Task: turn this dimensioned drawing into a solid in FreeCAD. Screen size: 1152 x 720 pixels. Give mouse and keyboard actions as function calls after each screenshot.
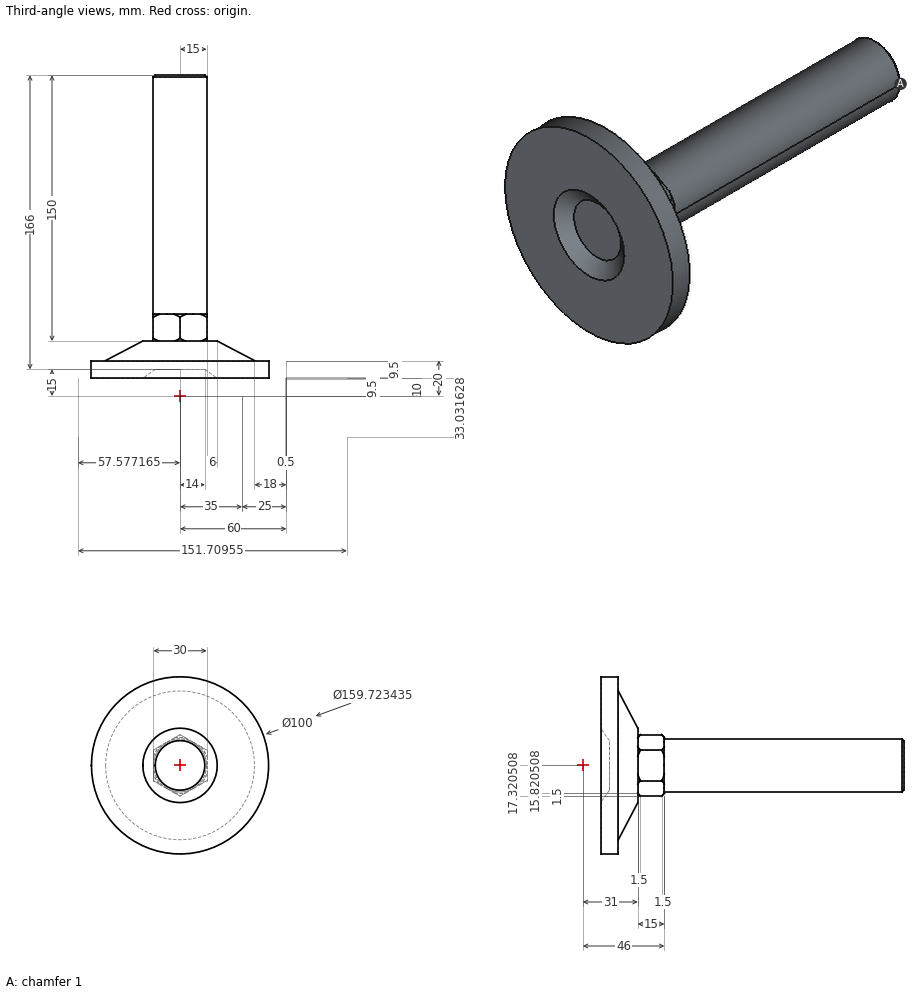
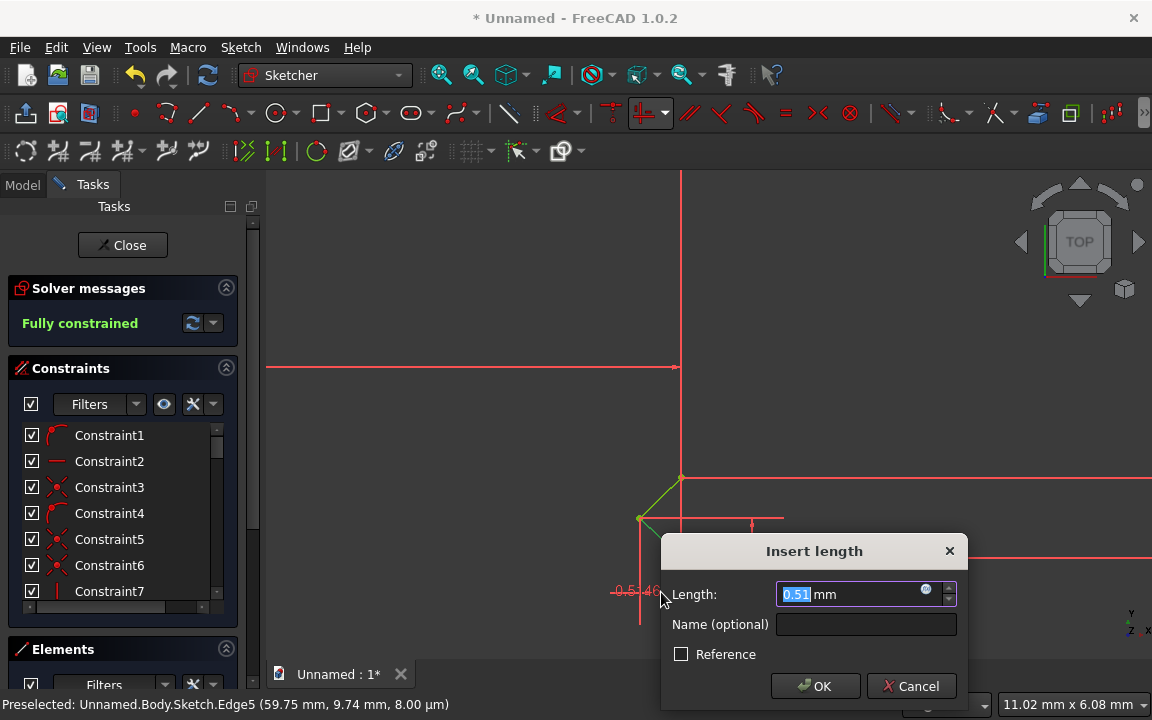
text(0.5)
key(Return)
key(Escape)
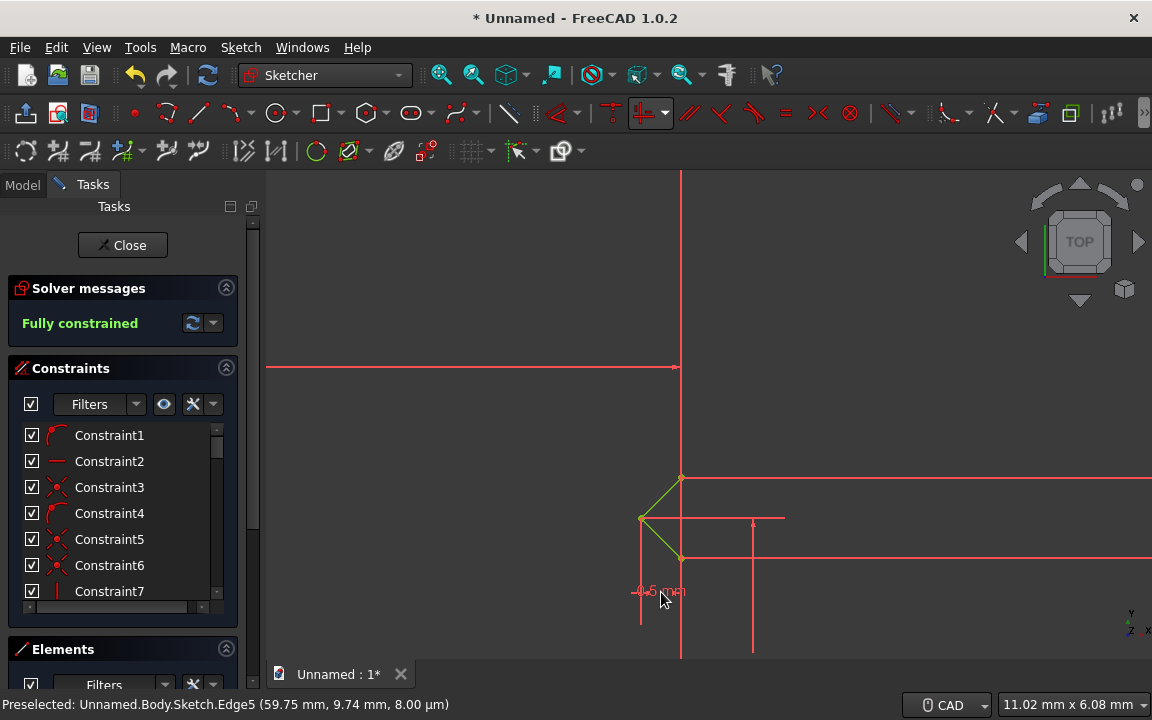
click(123, 245)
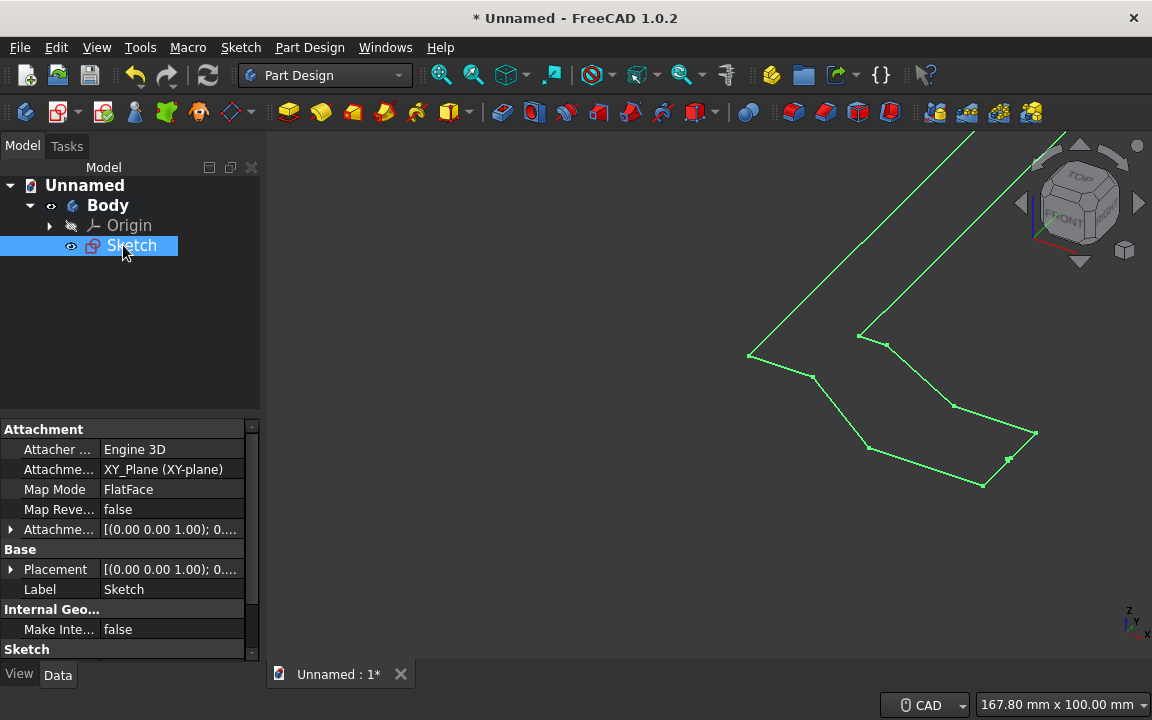
click(322, 112)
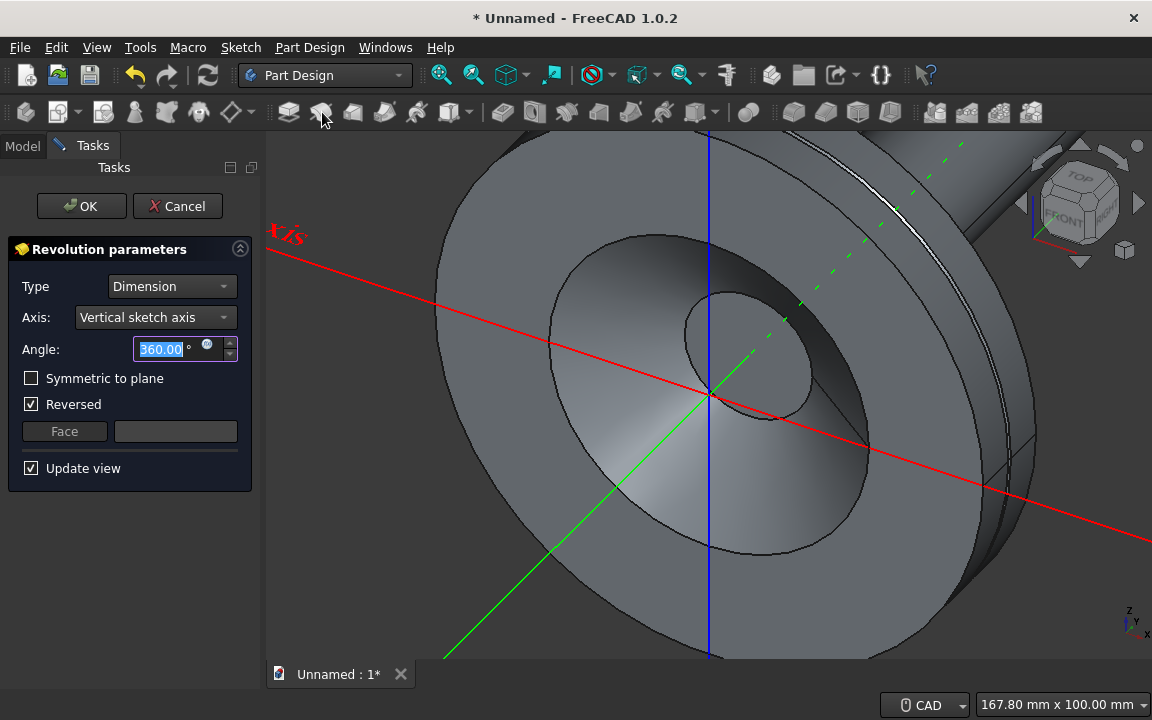
click(82, 206)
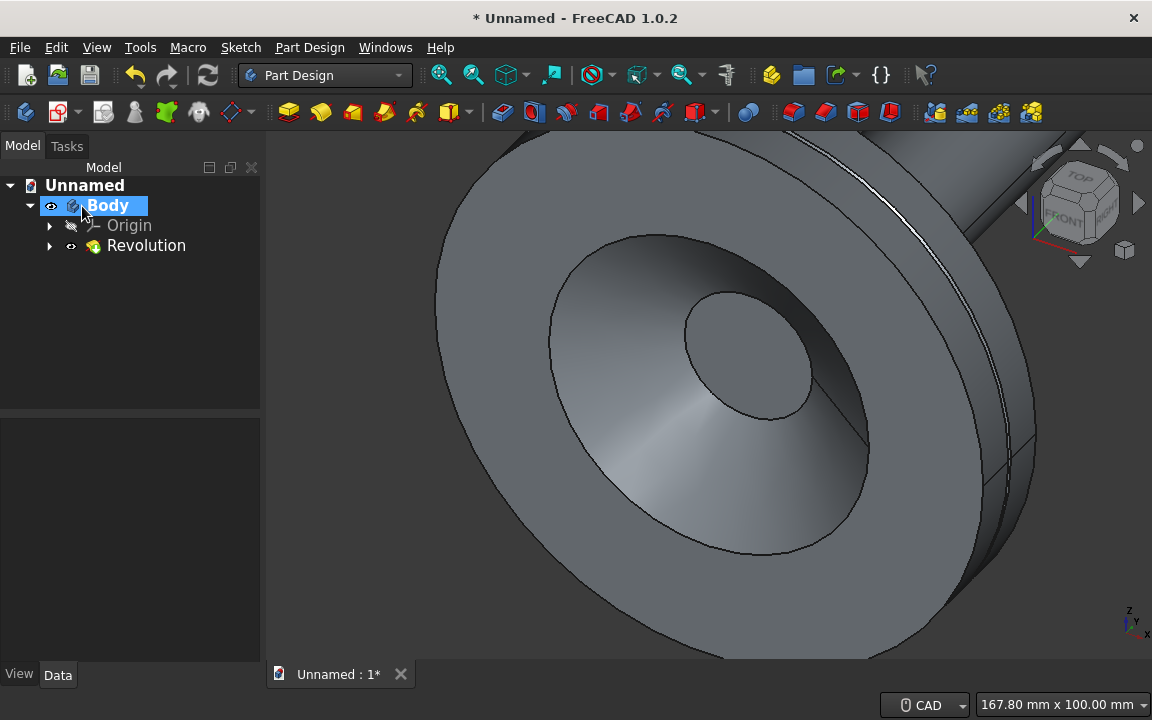
click(442, 76)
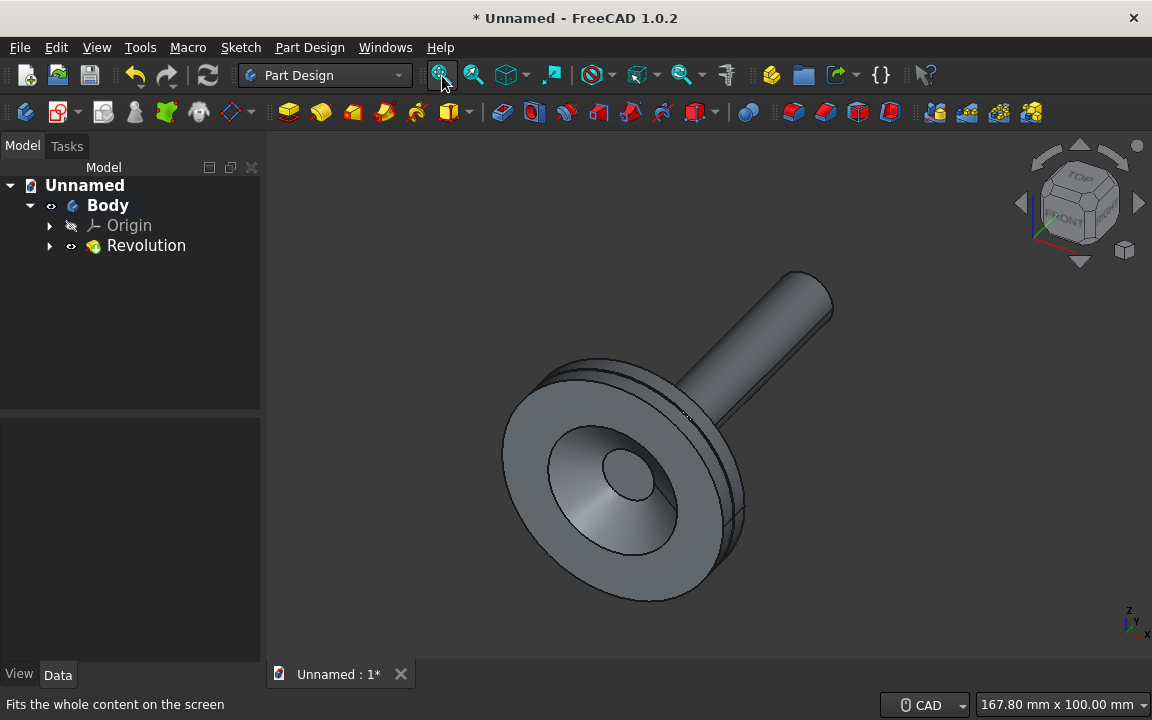
key(4)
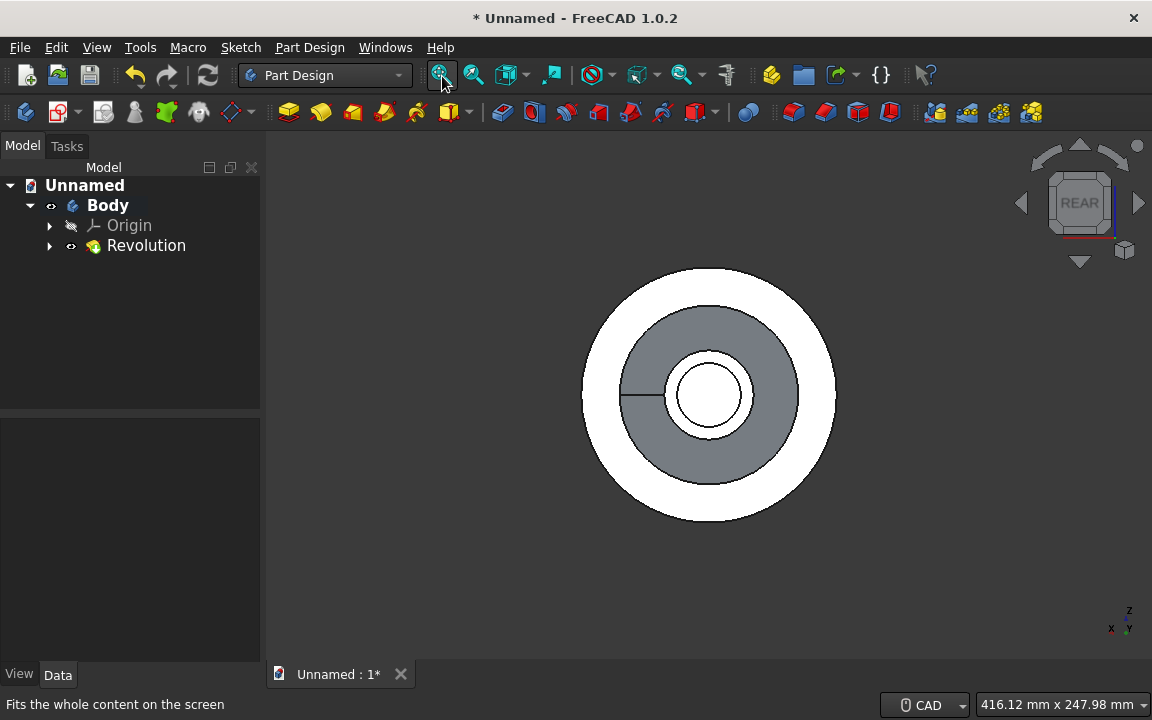
scroll(671, 394, up, 4)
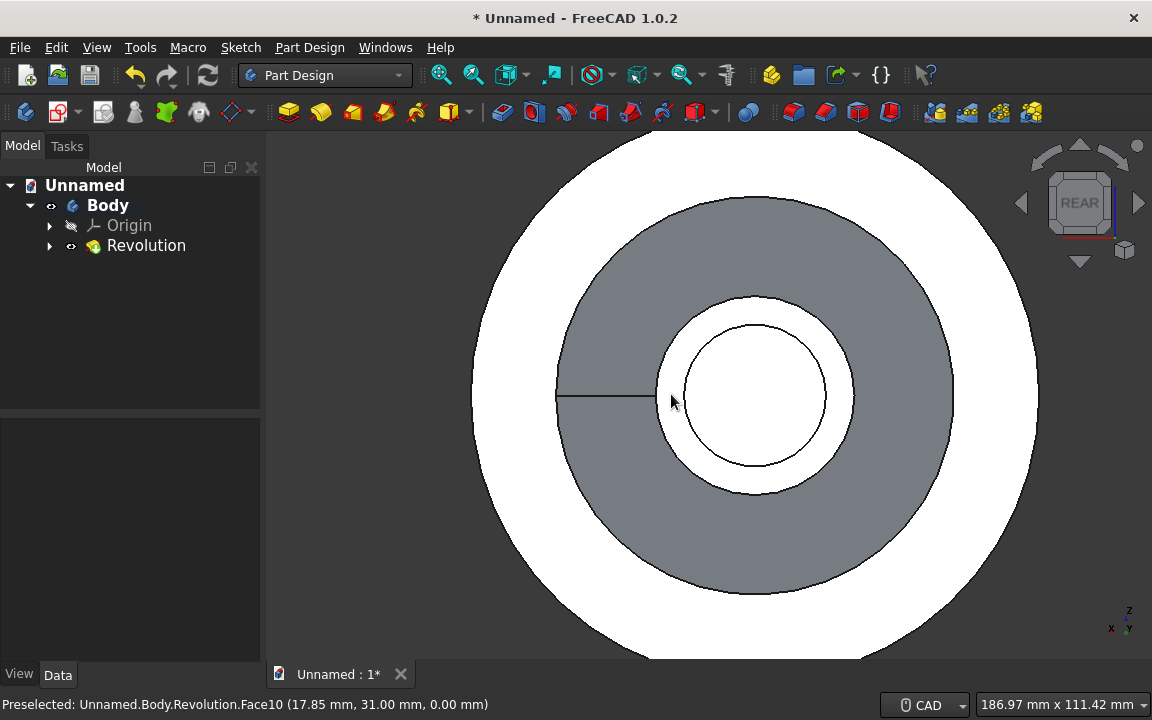
click(670, 395)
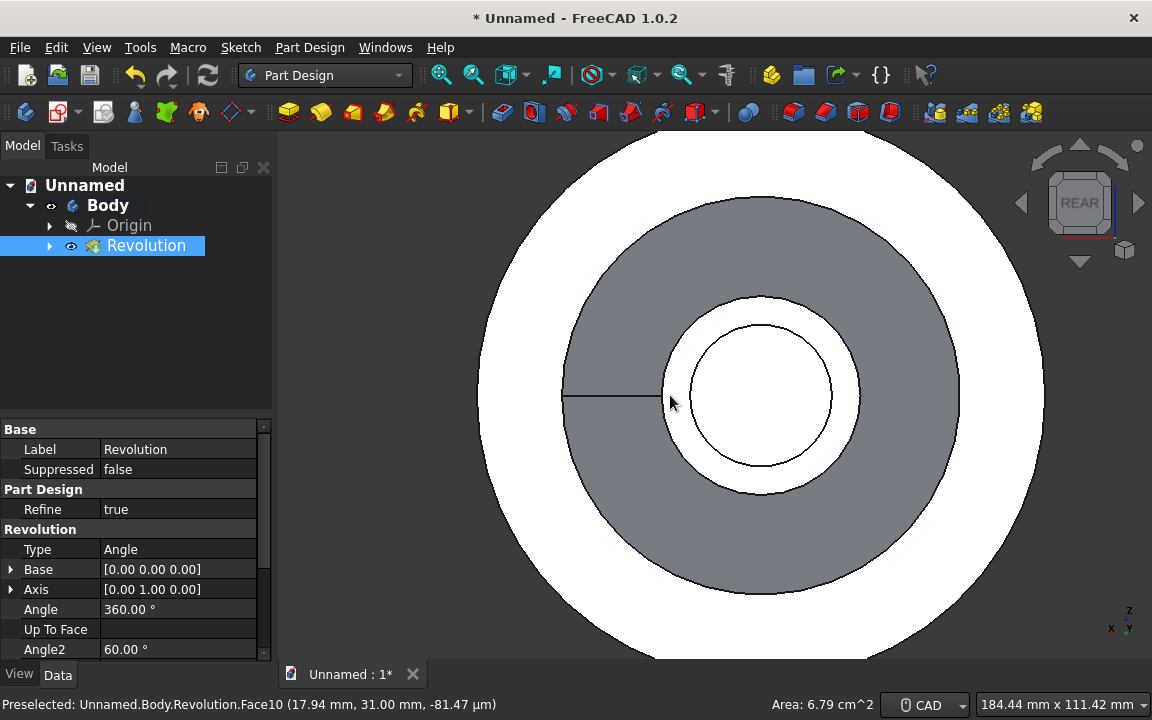
click(58, 112)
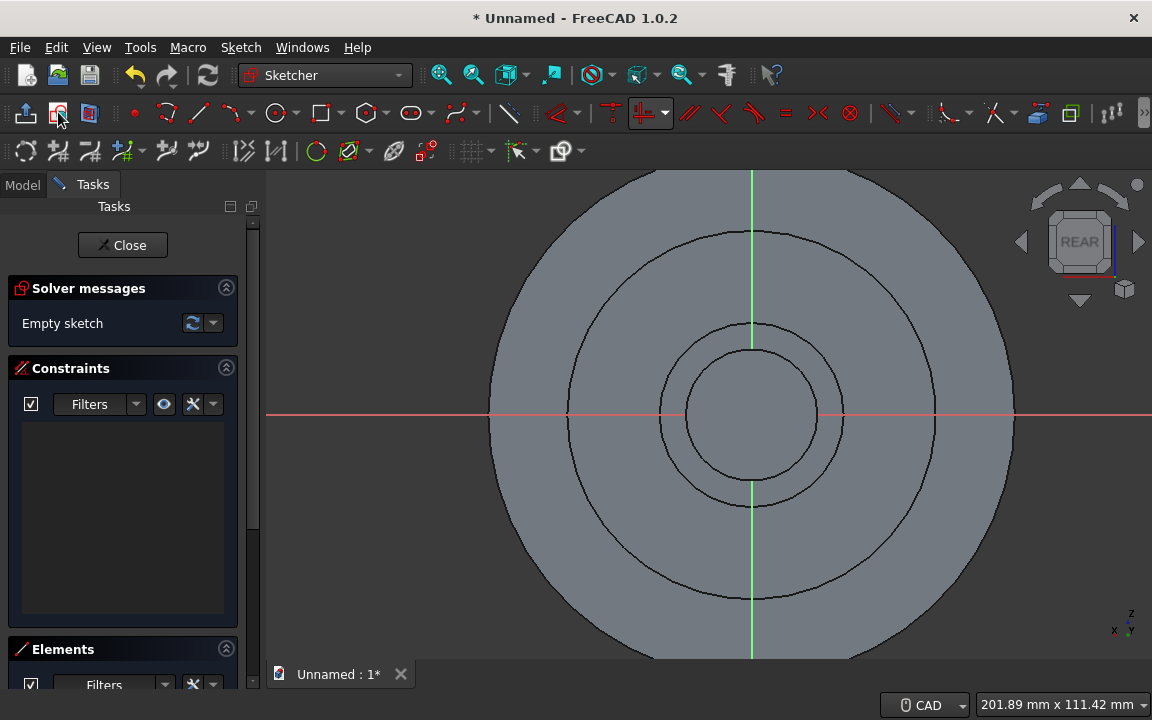
scroll(887, 416, up, 3)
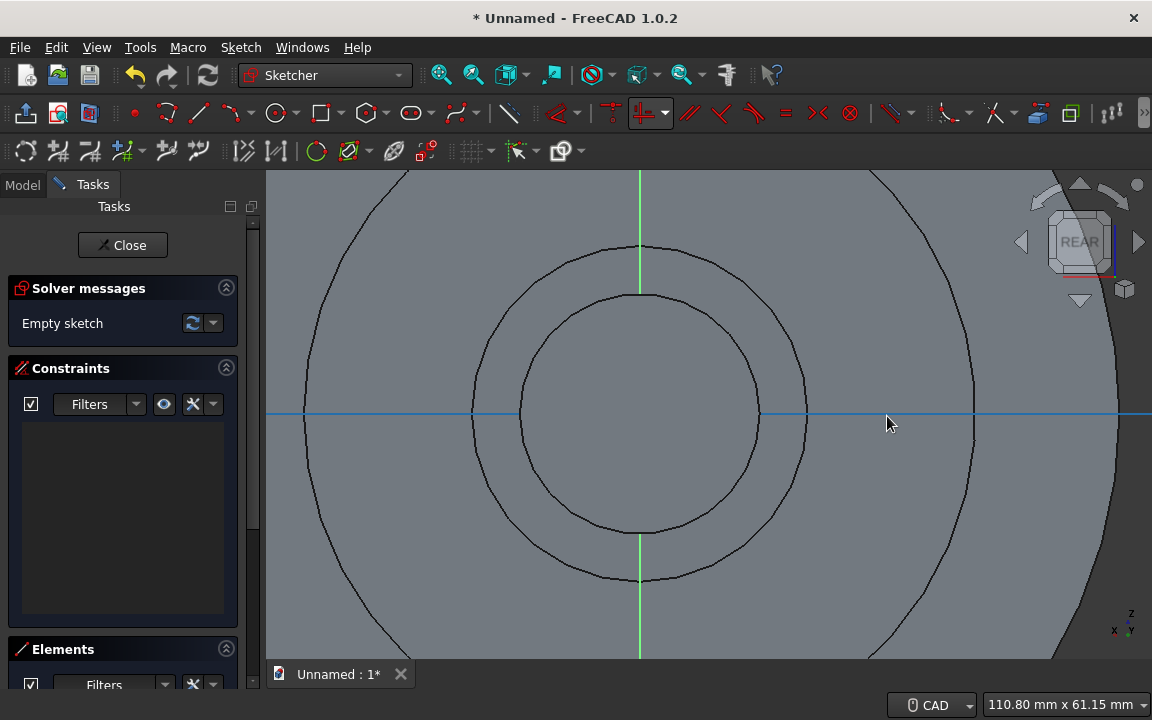
click(366, 114)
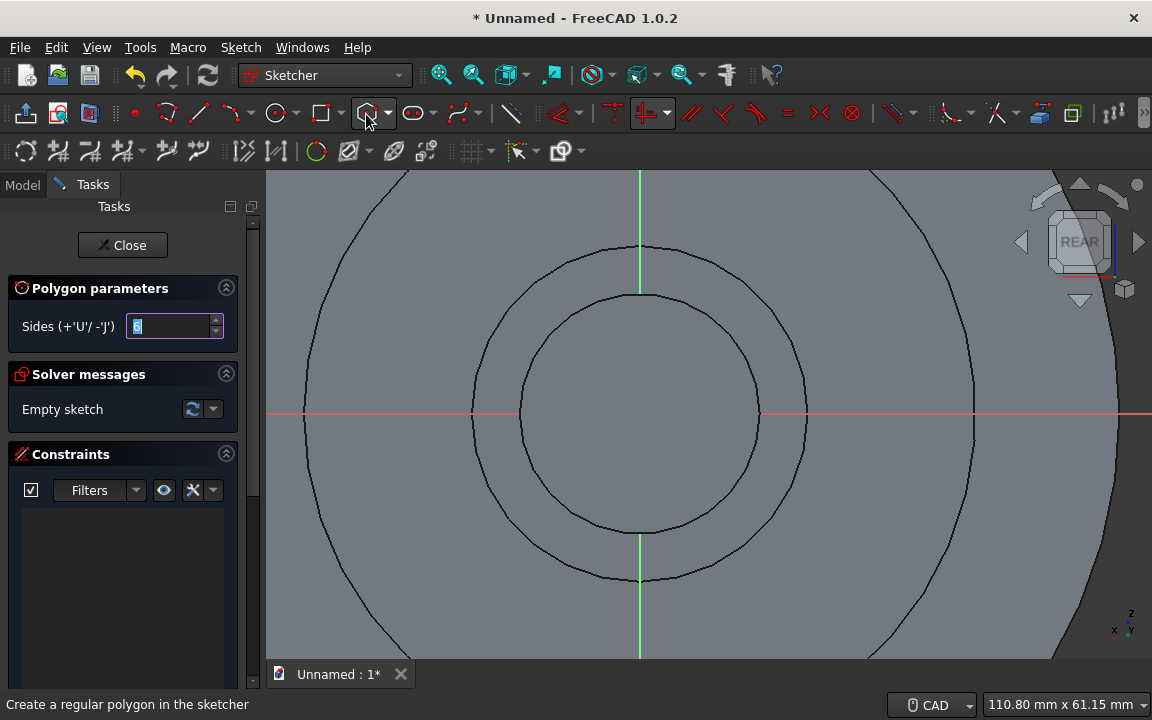
click(640, 414)